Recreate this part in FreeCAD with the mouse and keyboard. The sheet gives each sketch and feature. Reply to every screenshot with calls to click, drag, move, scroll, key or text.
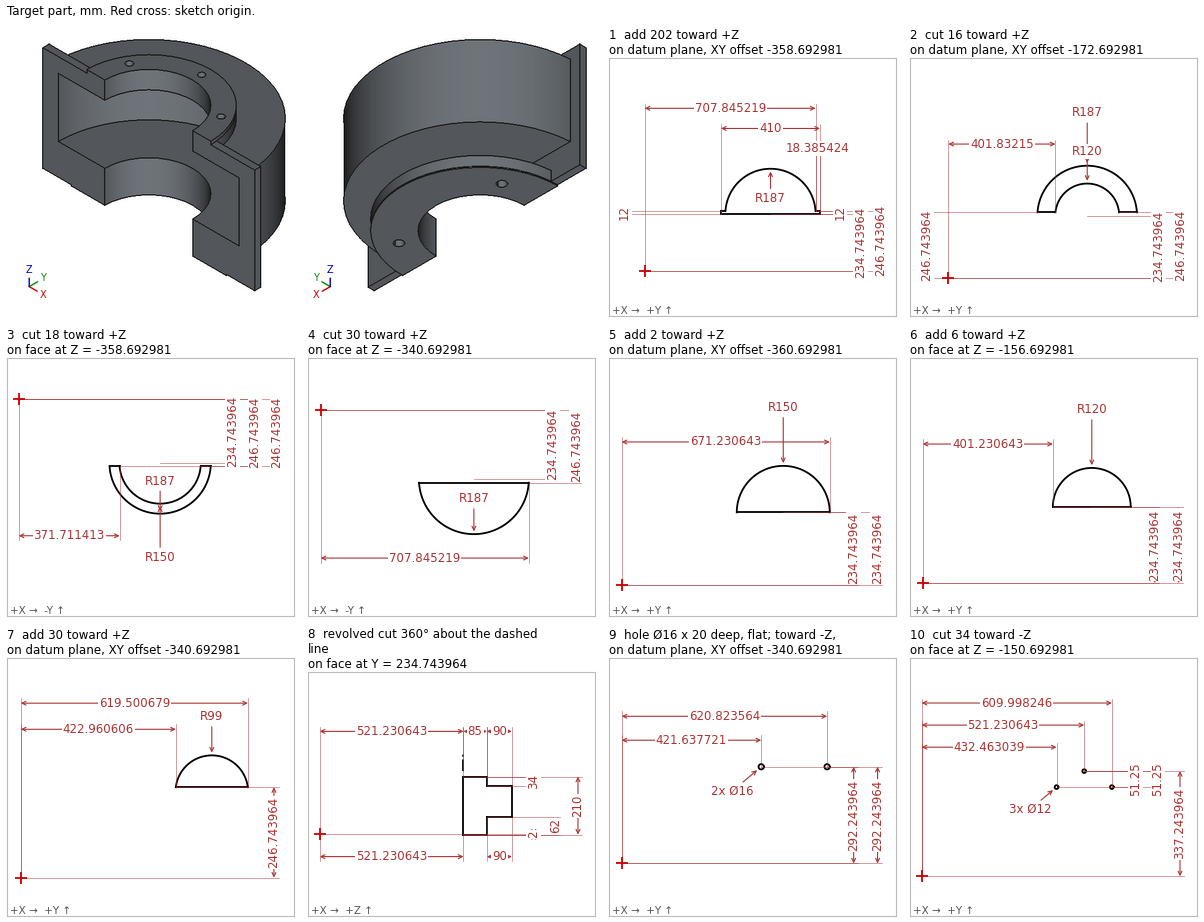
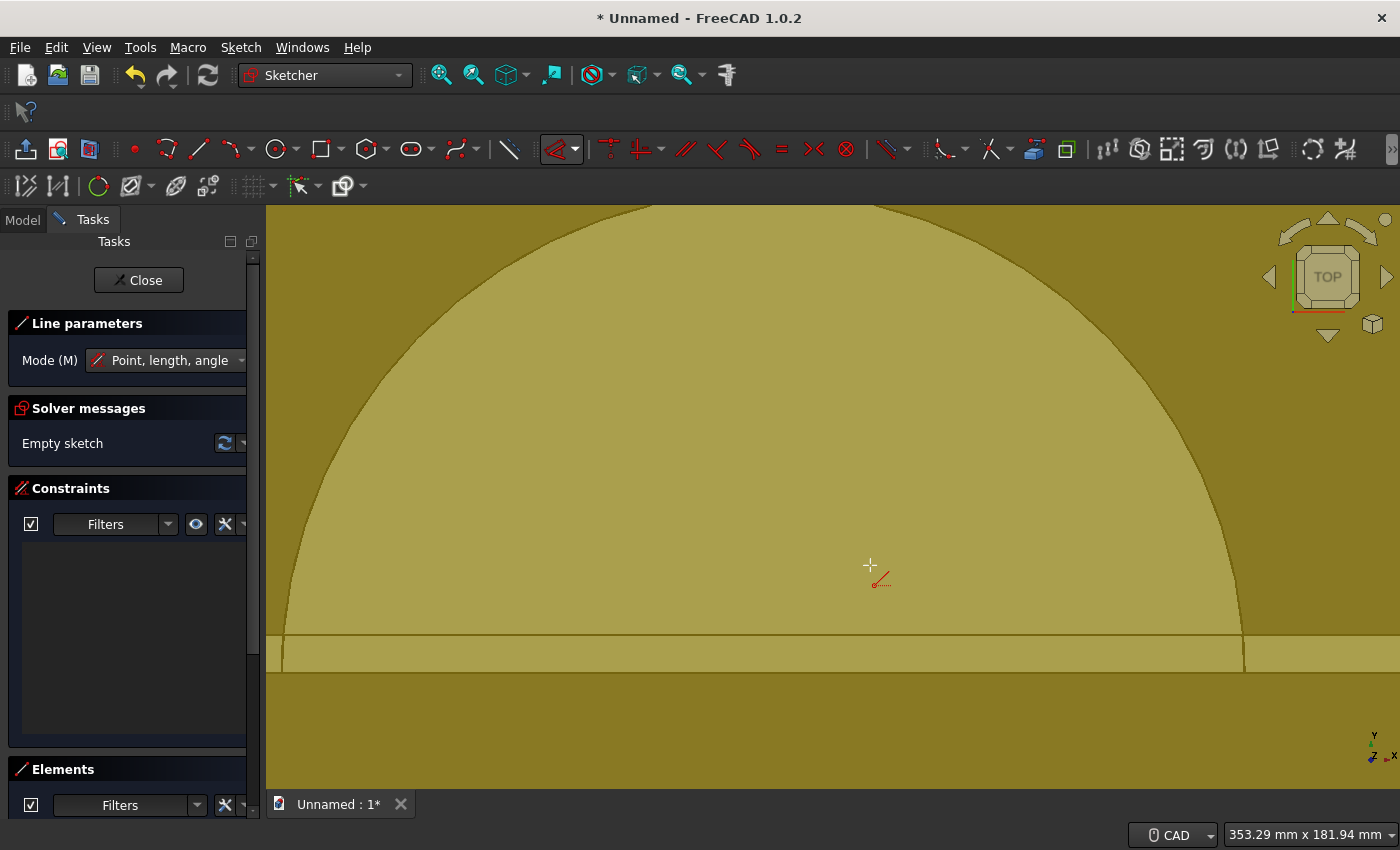
click(448, 635)
click(1079, 635)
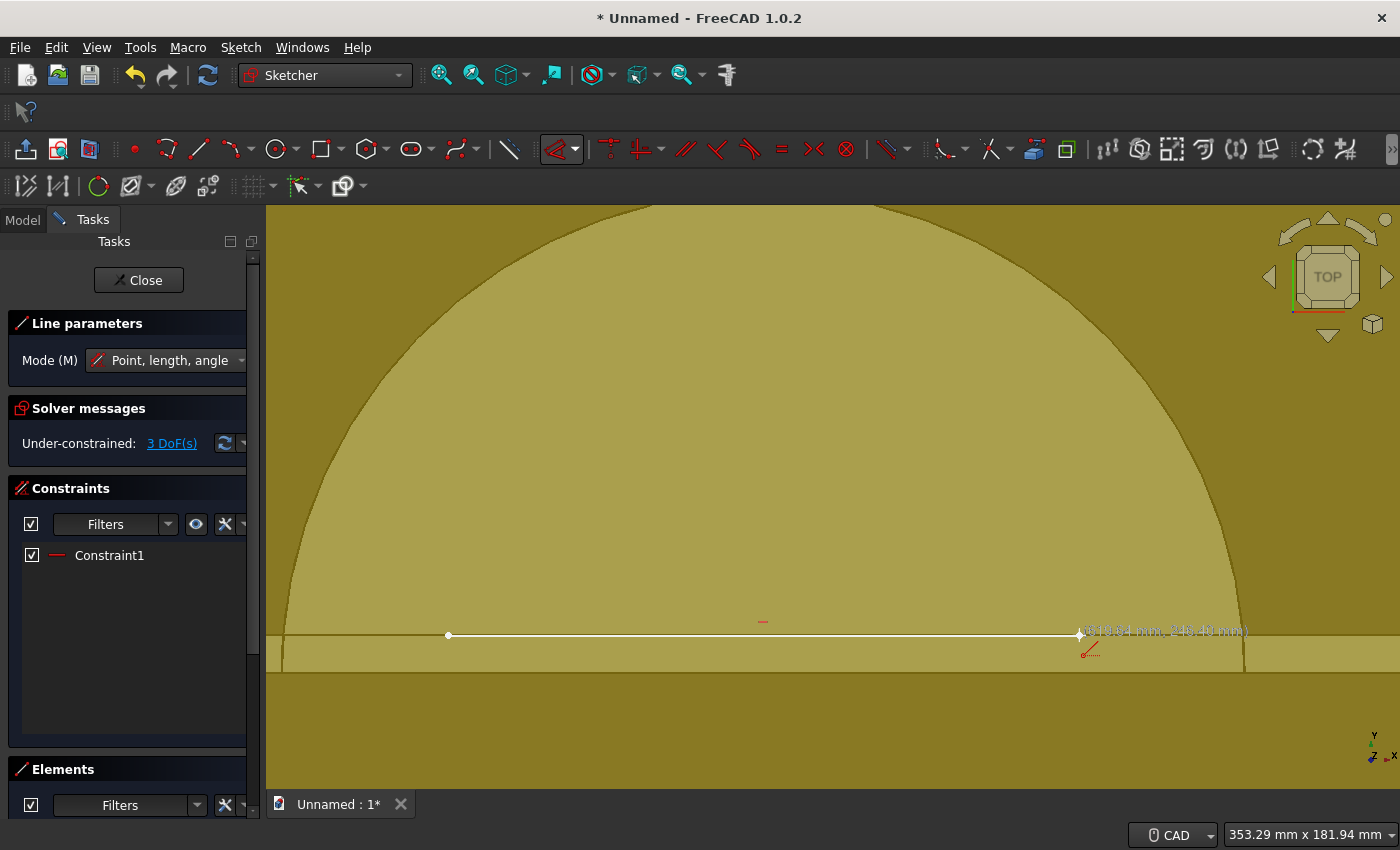
key(g)
key(3)
key(a)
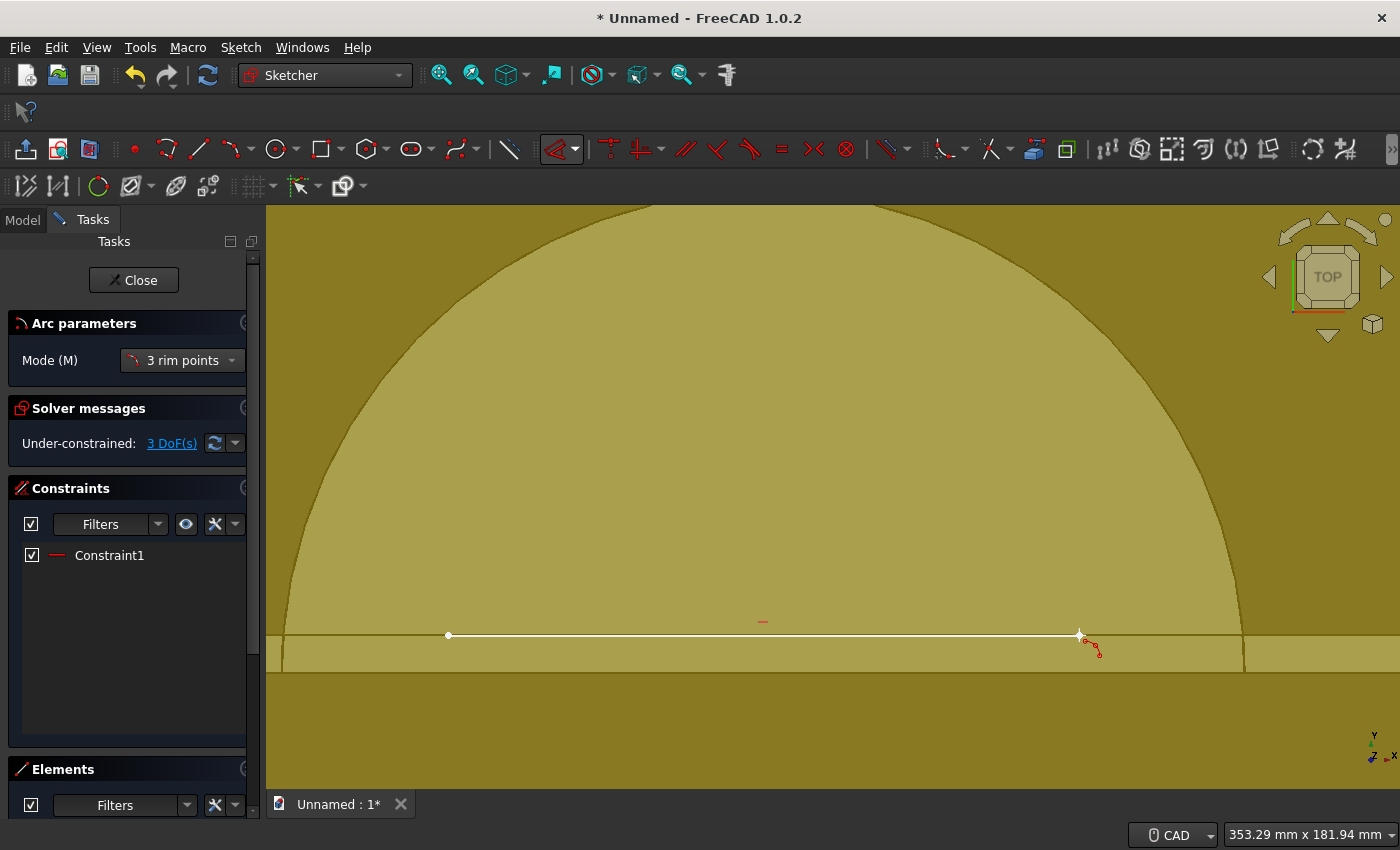
click(1079, 636)
click(448, 636)
click(763, 356)
key(Escape)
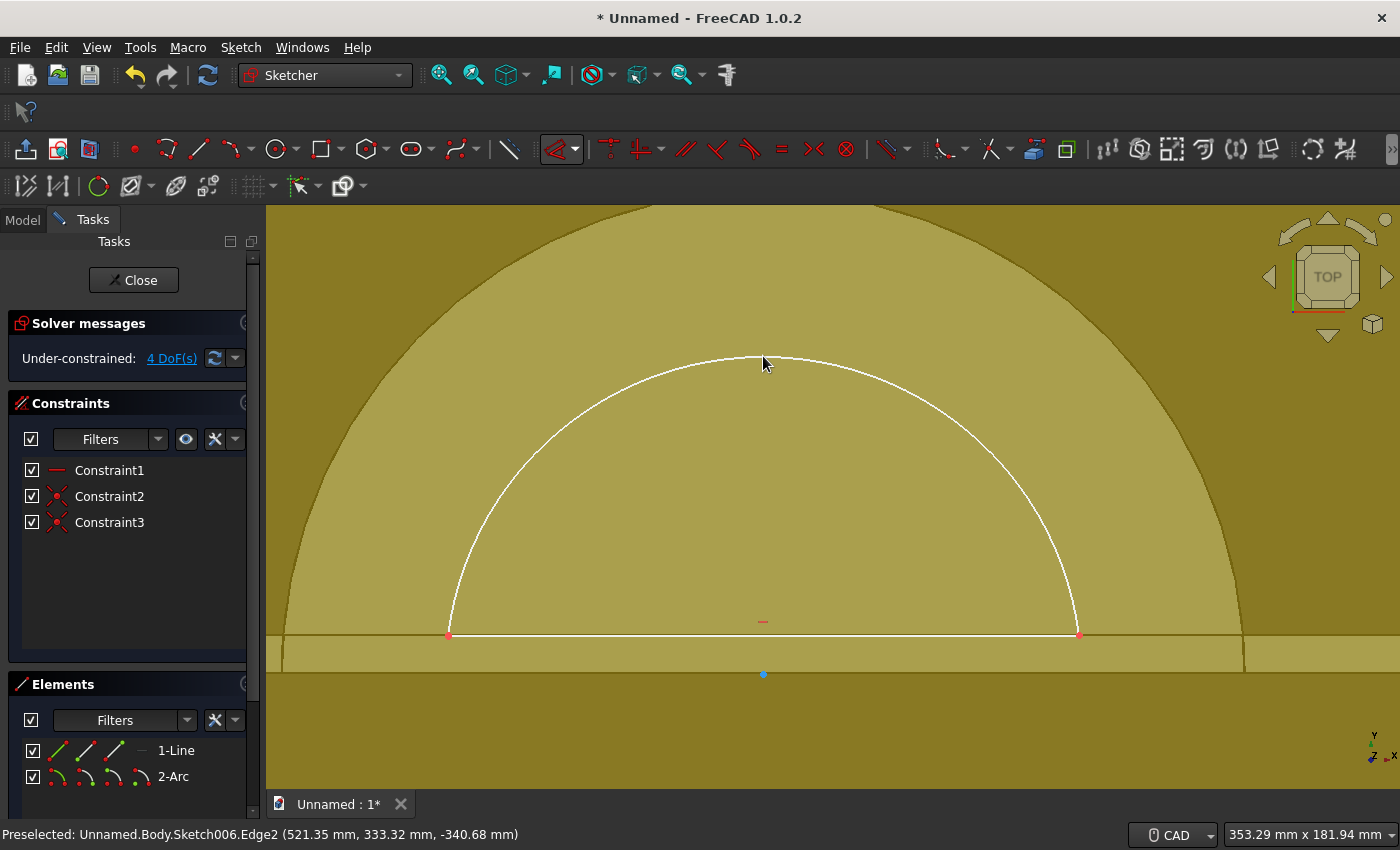
key(d)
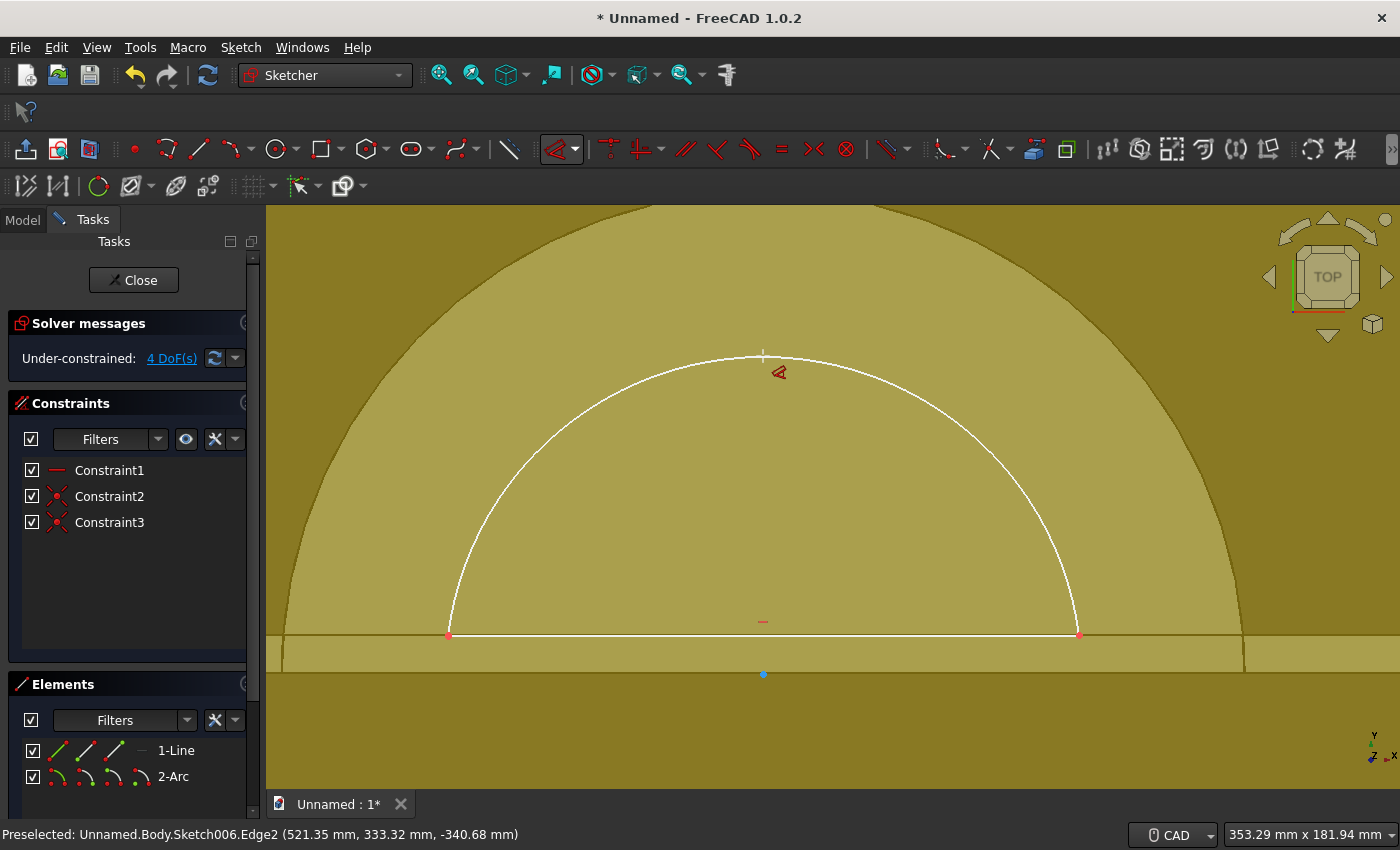
click(938, 409)
click(956, 382)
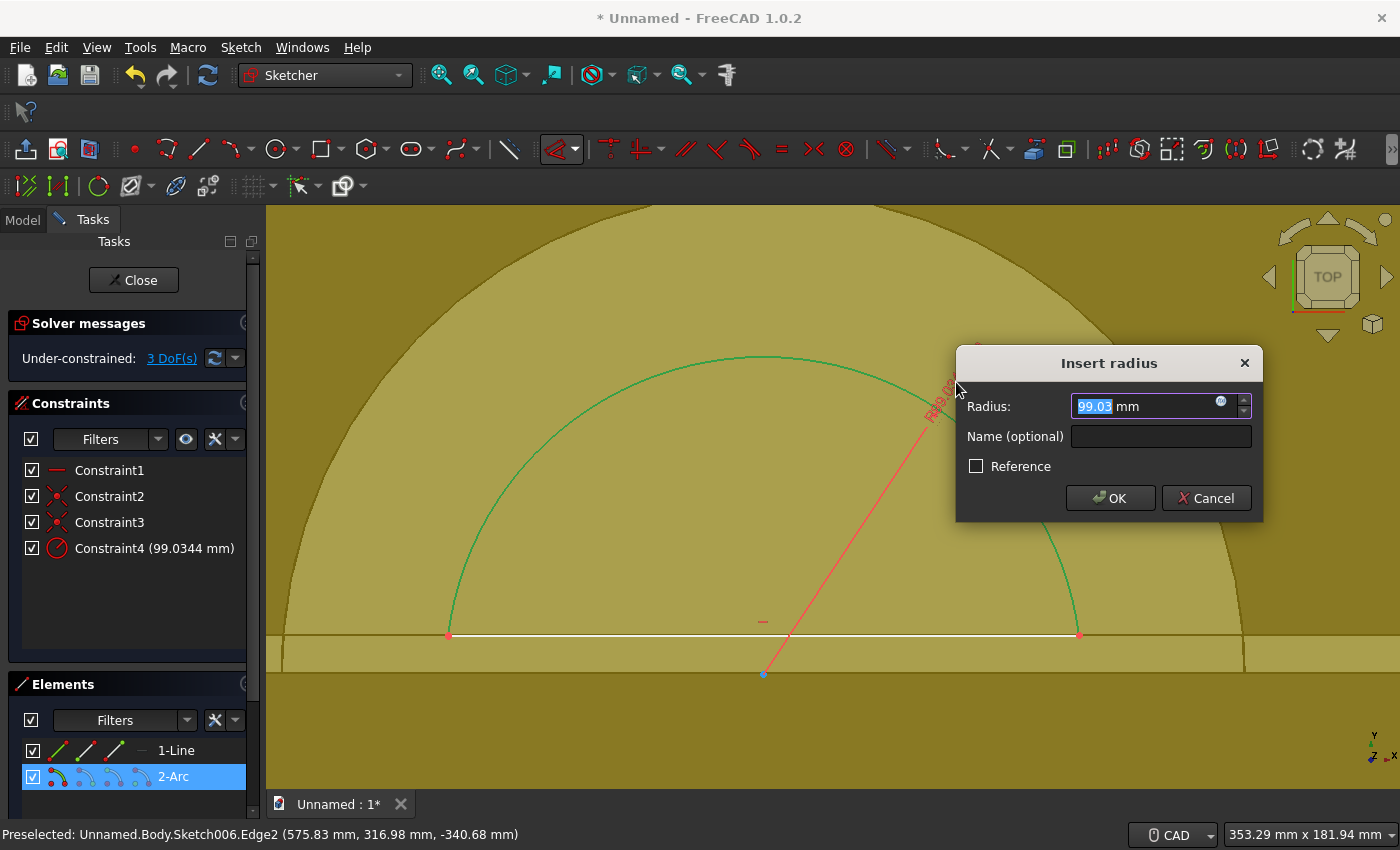
text(99)
key(Return)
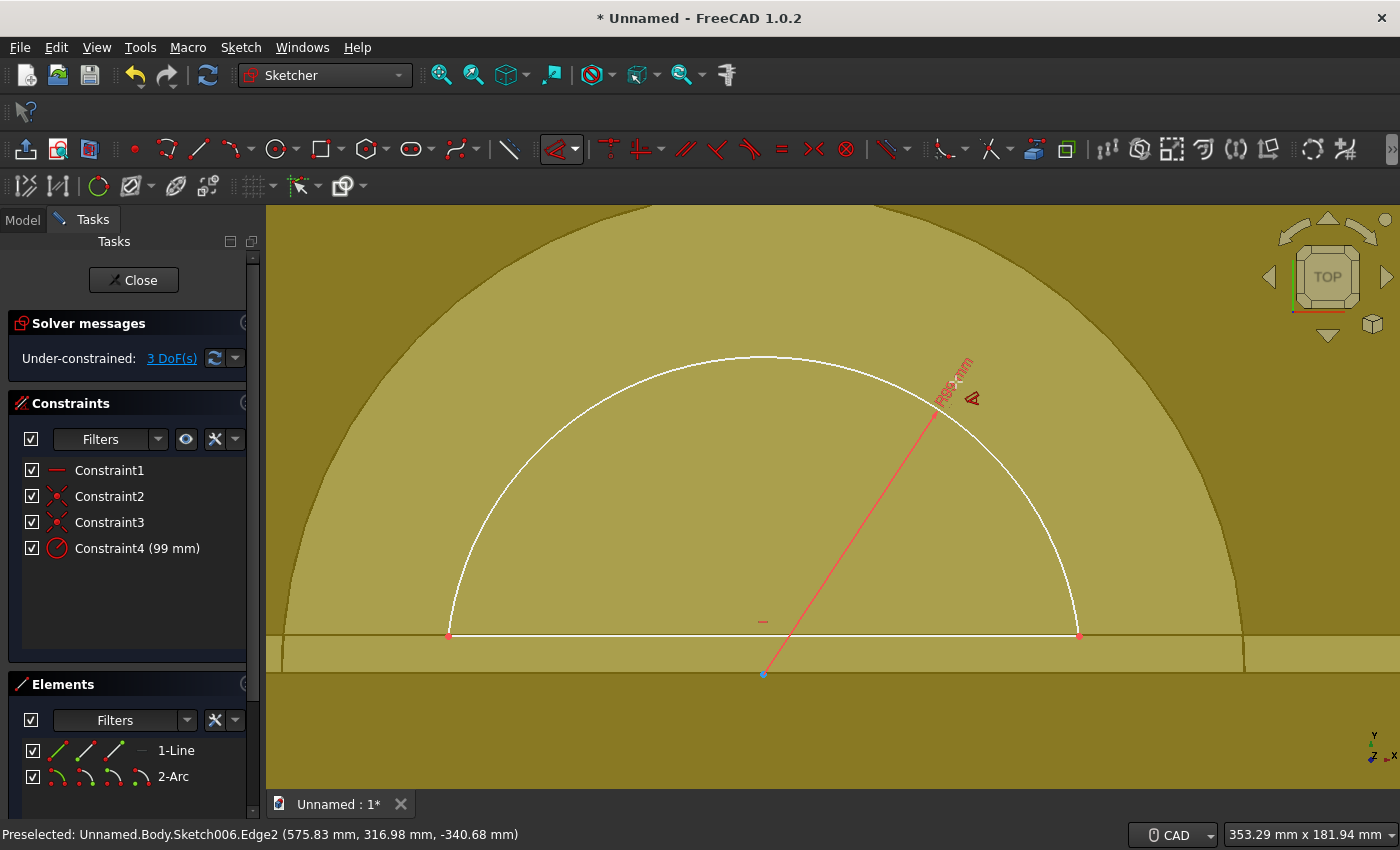
click(448, 636)
click(371, 602)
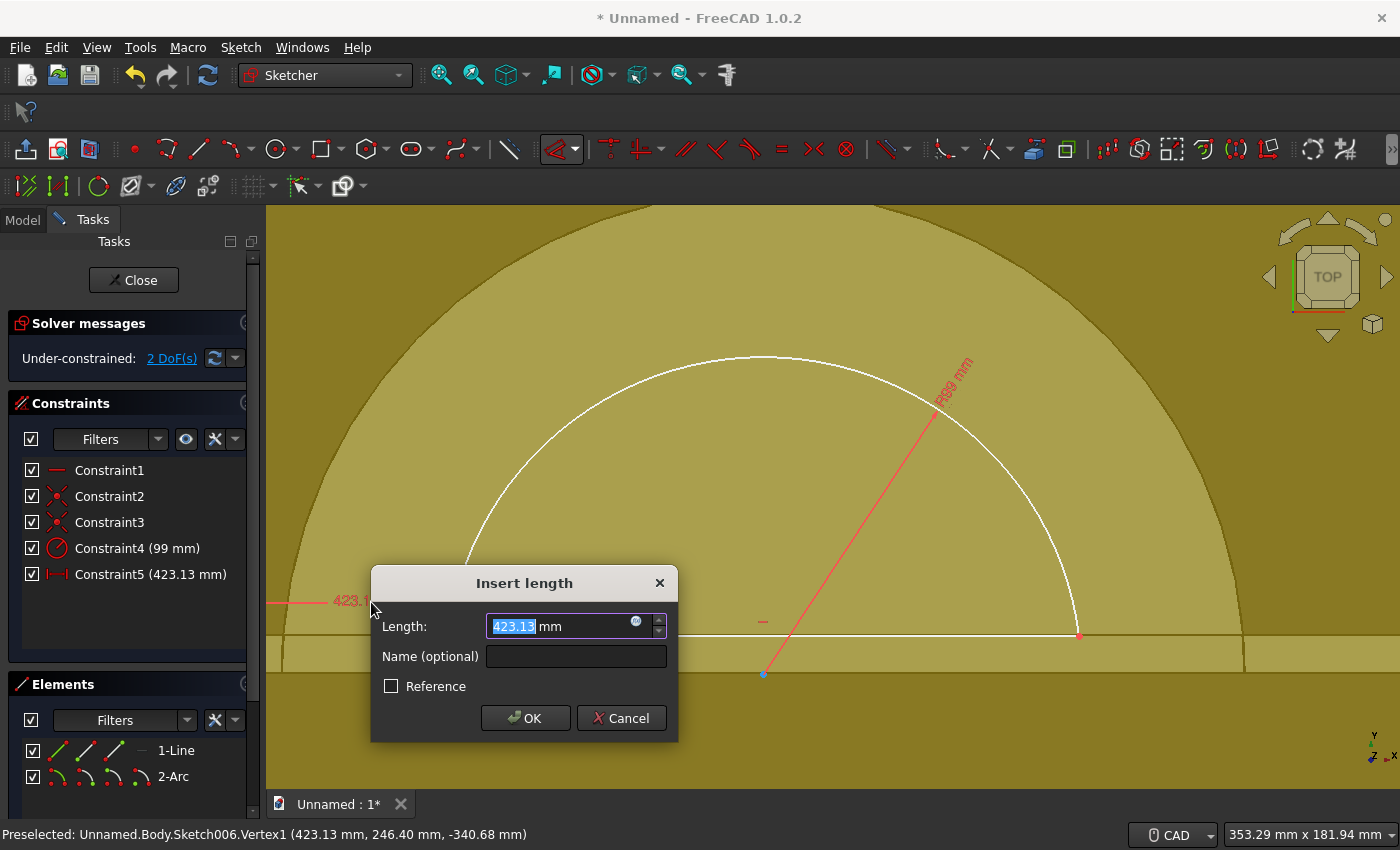
text(422.960606)
key(Return)